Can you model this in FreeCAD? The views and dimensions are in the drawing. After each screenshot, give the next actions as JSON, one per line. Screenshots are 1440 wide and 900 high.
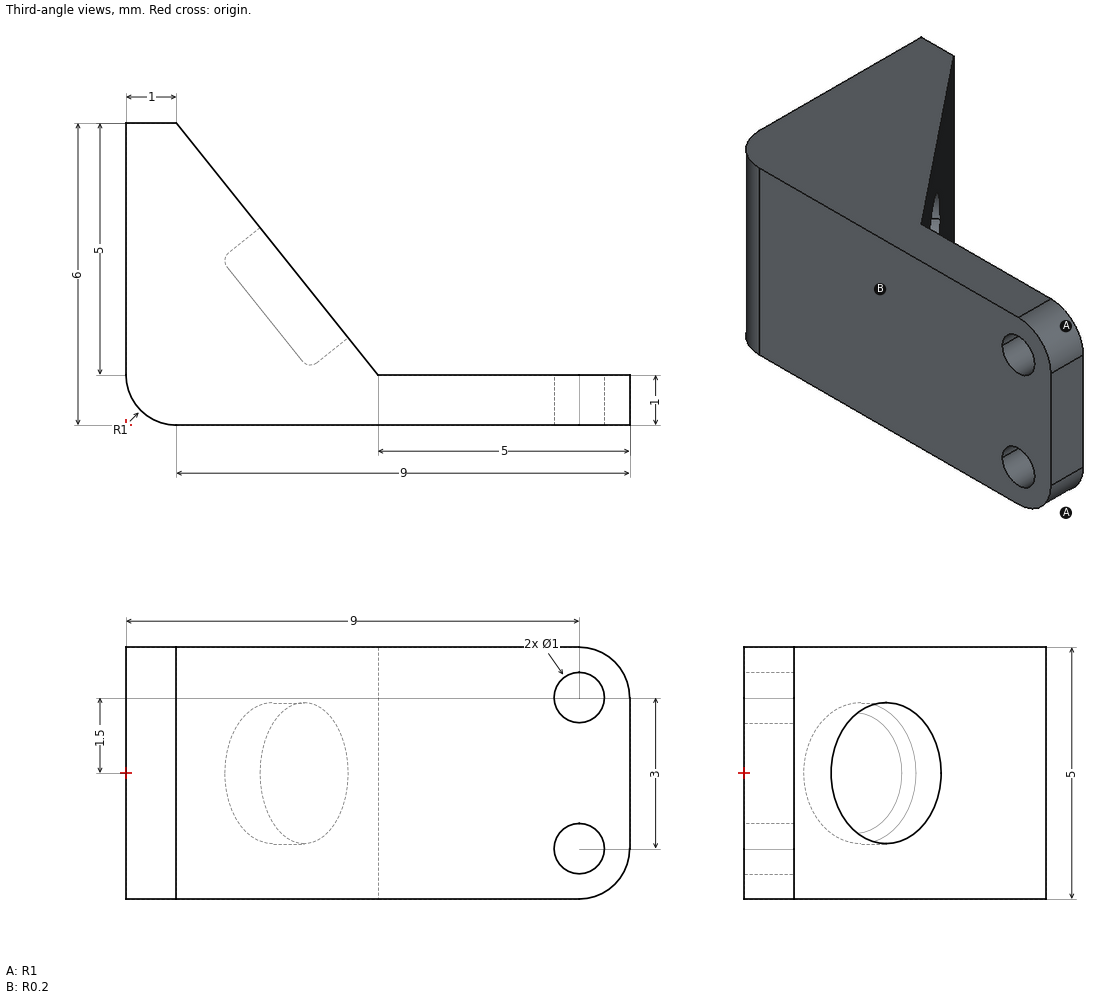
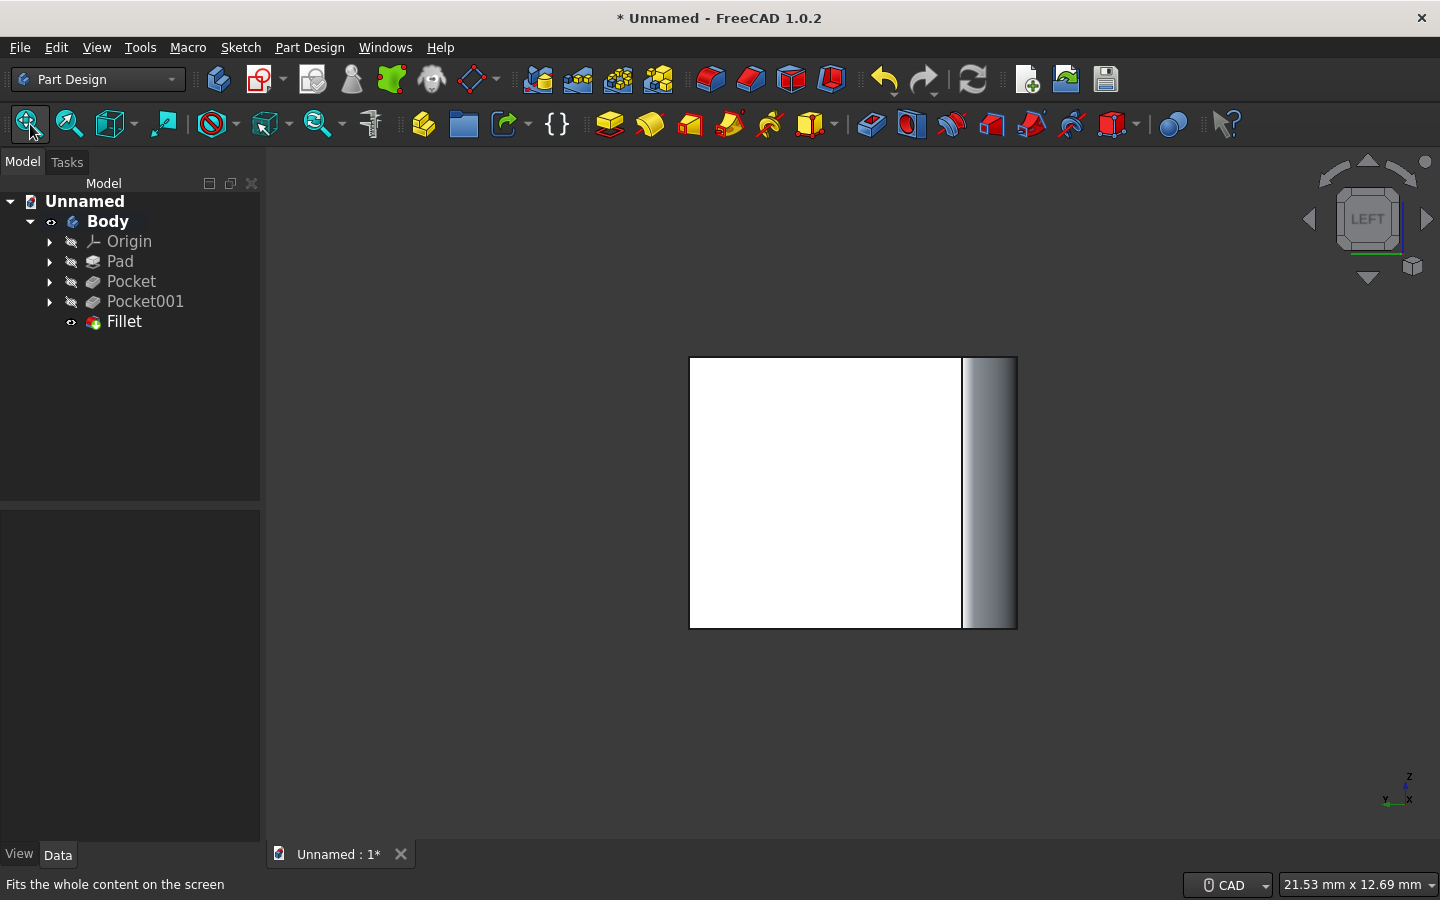
{"action": "key", "text": "v f"}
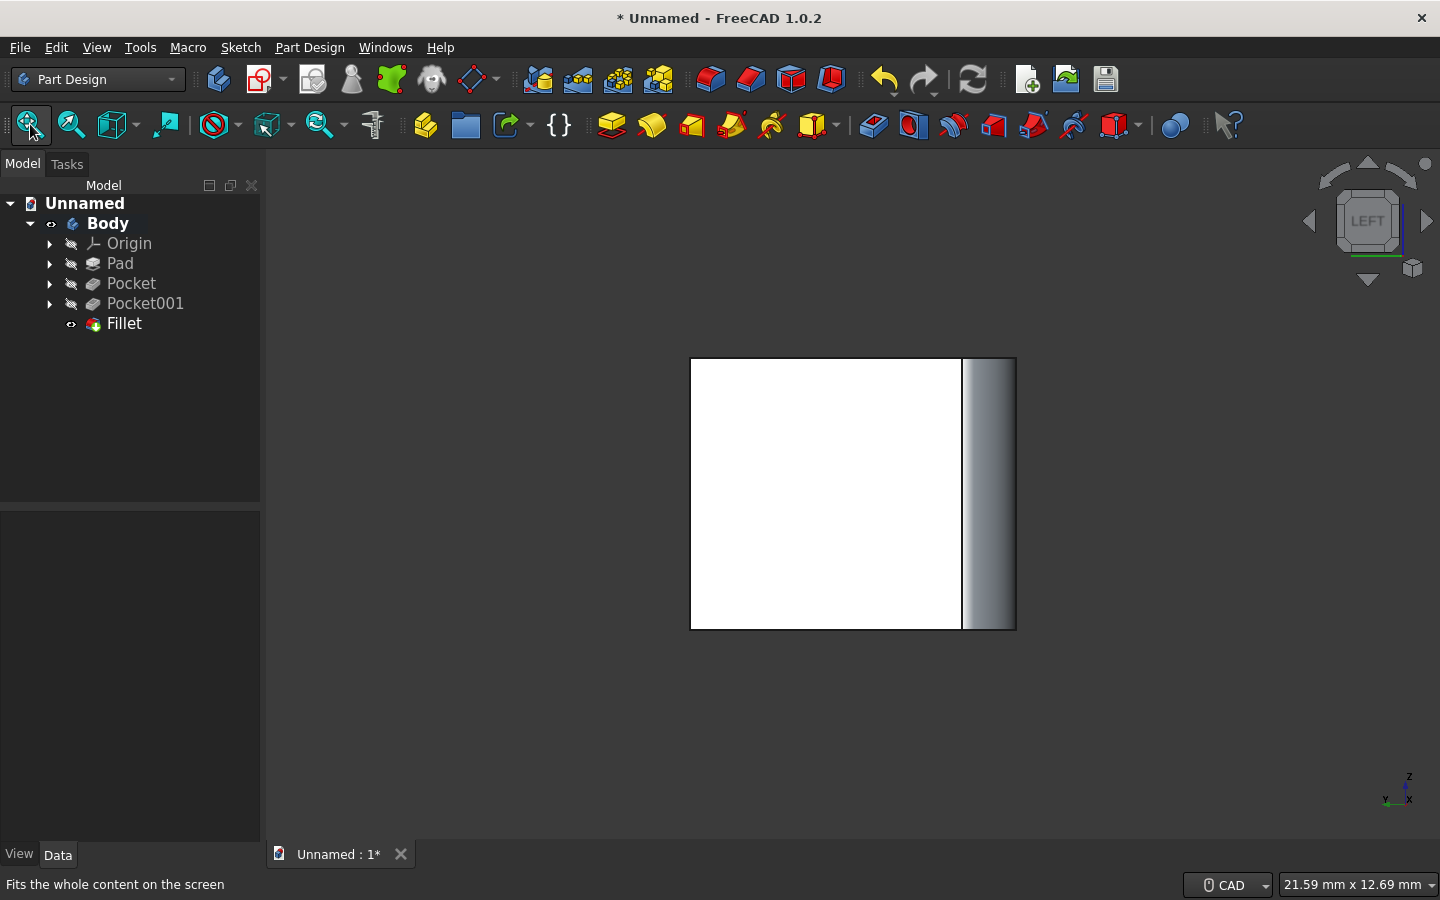
{"action": "key", "text": "v 3"}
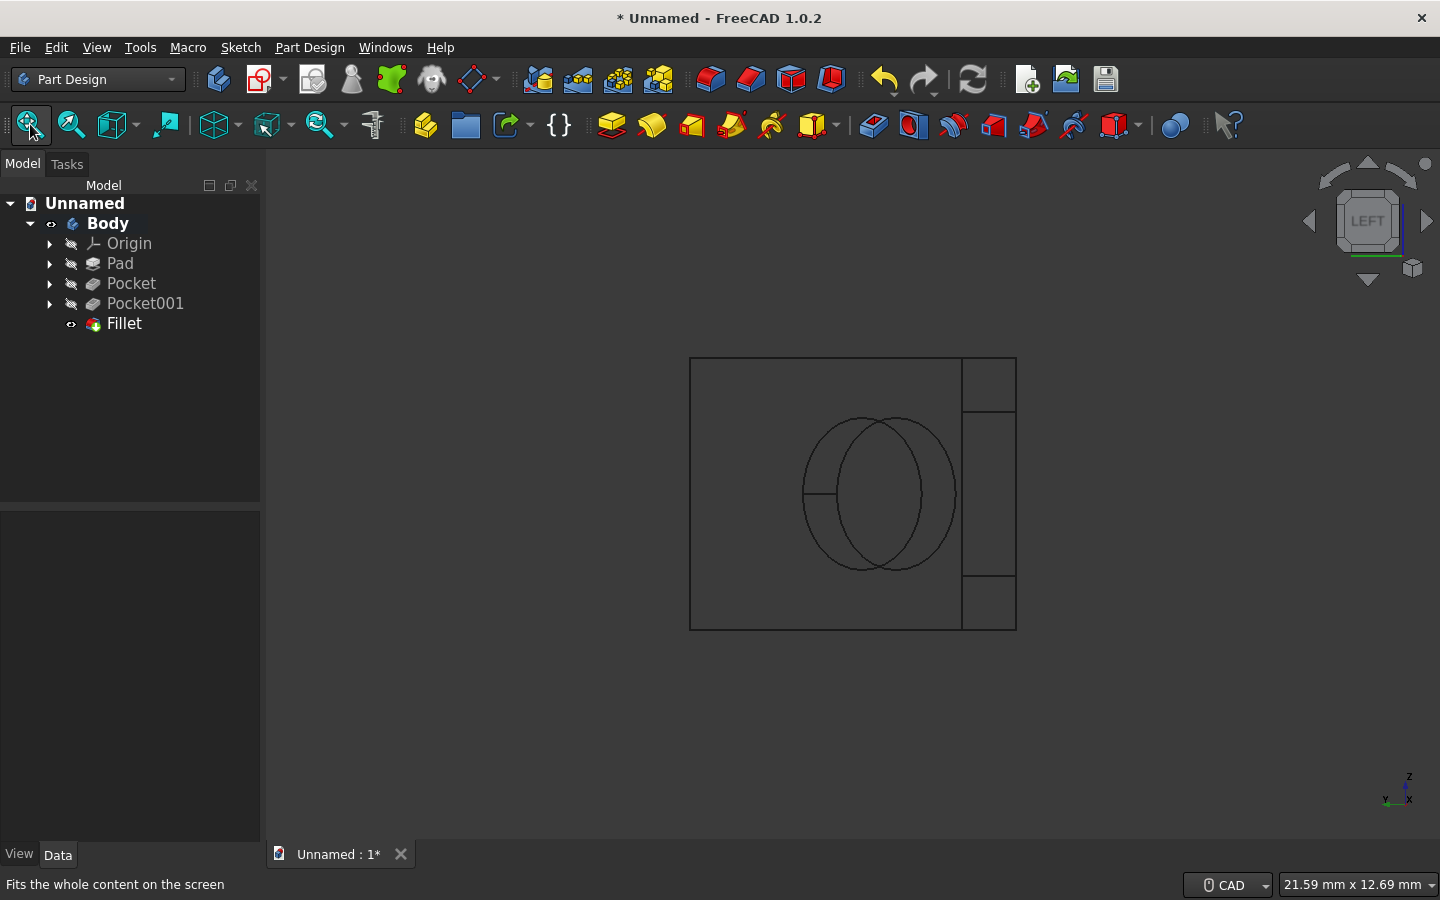
{"action": "key", "text": "0"}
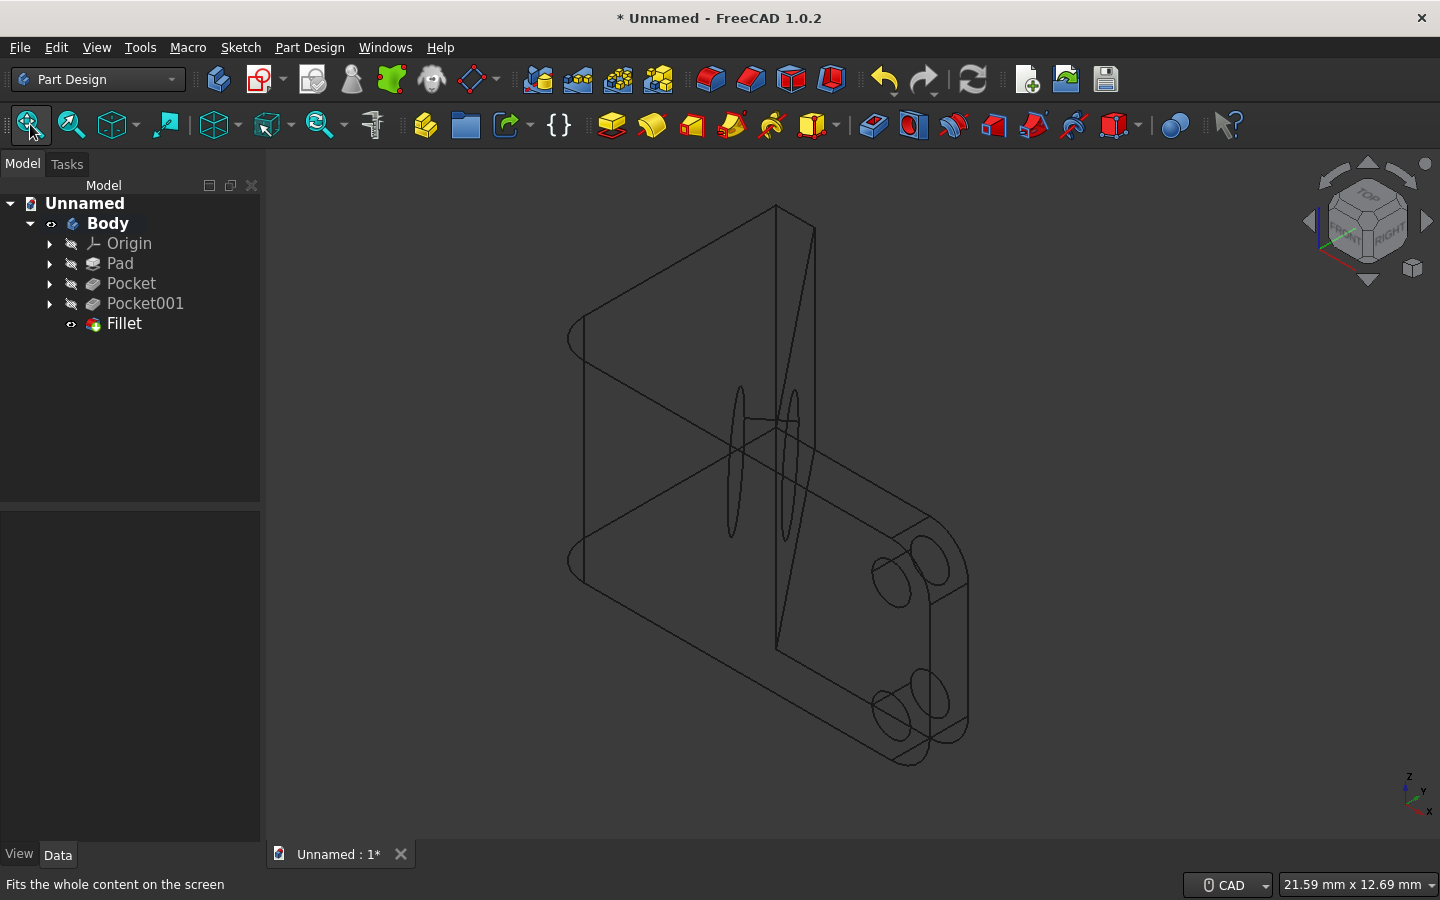
{"action": "left_click", "coordinate": [728, 505]}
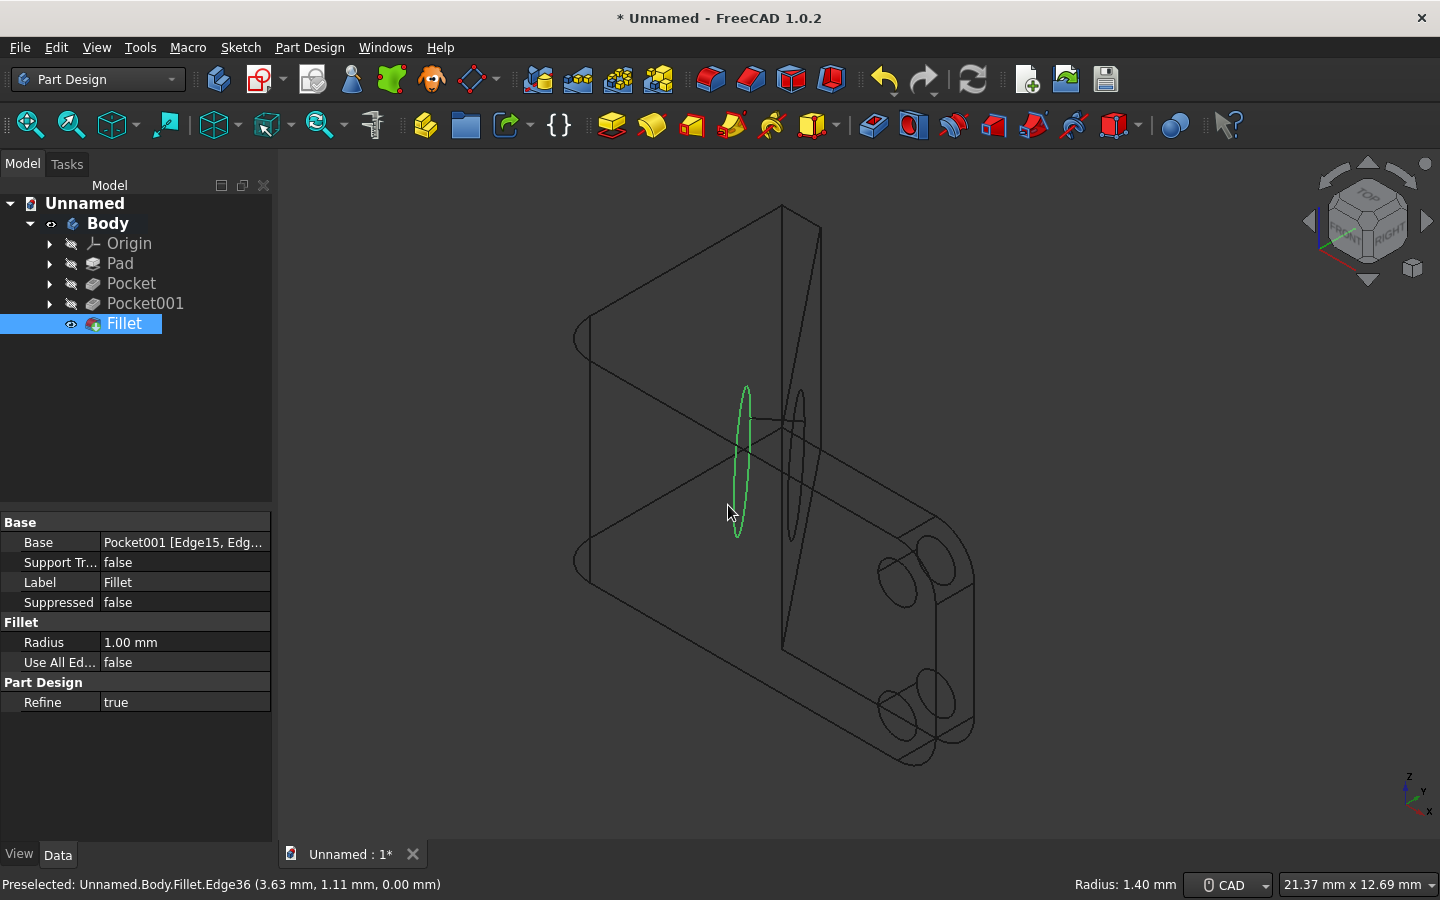
{"action": "key", "text": "v 1"}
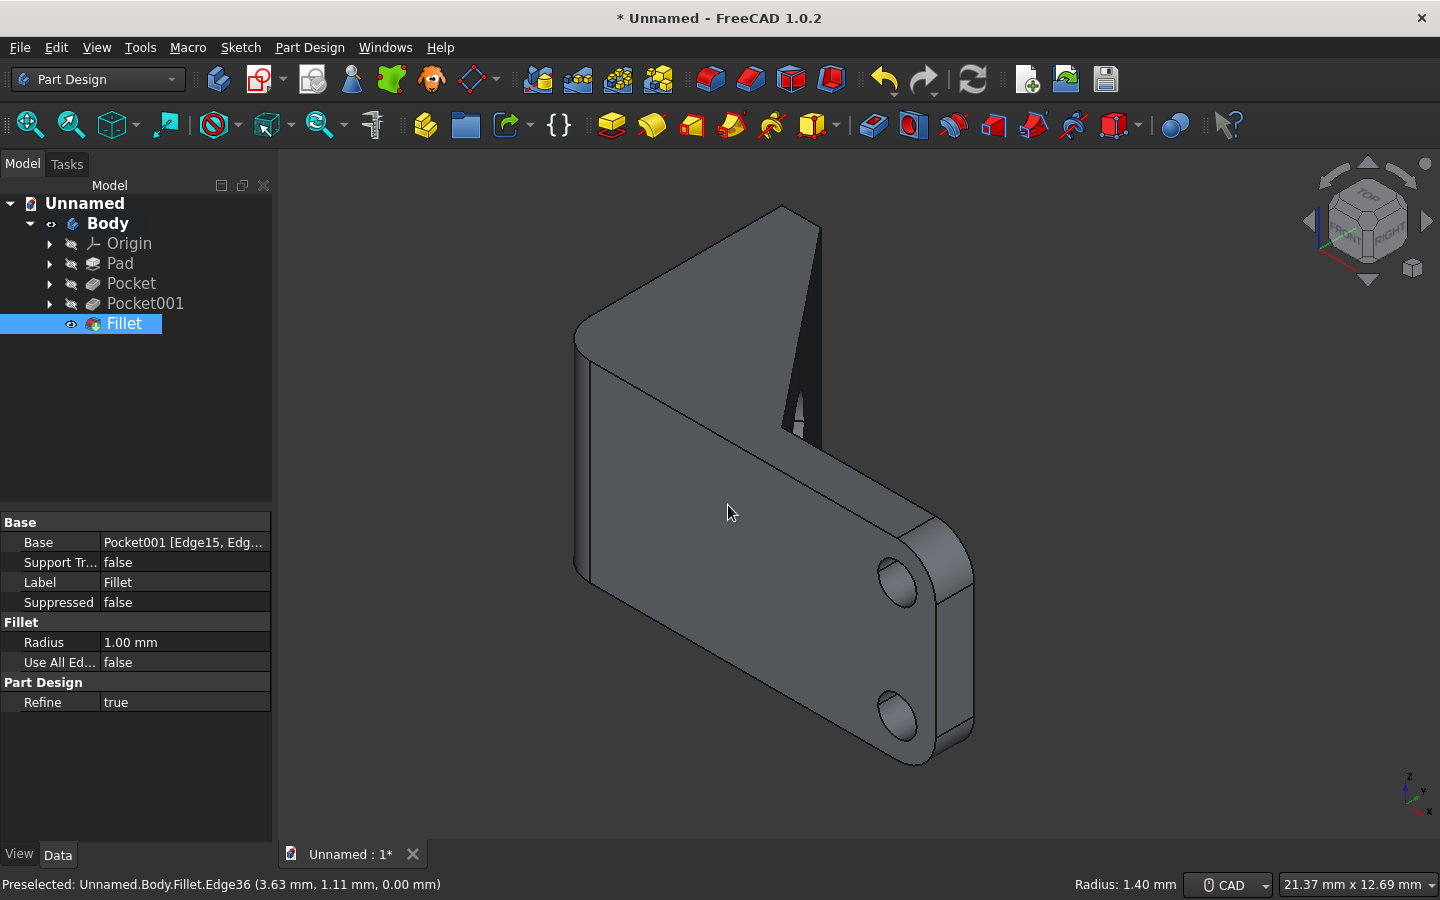
{"action": "left_click", "coordinate": [712, 80]}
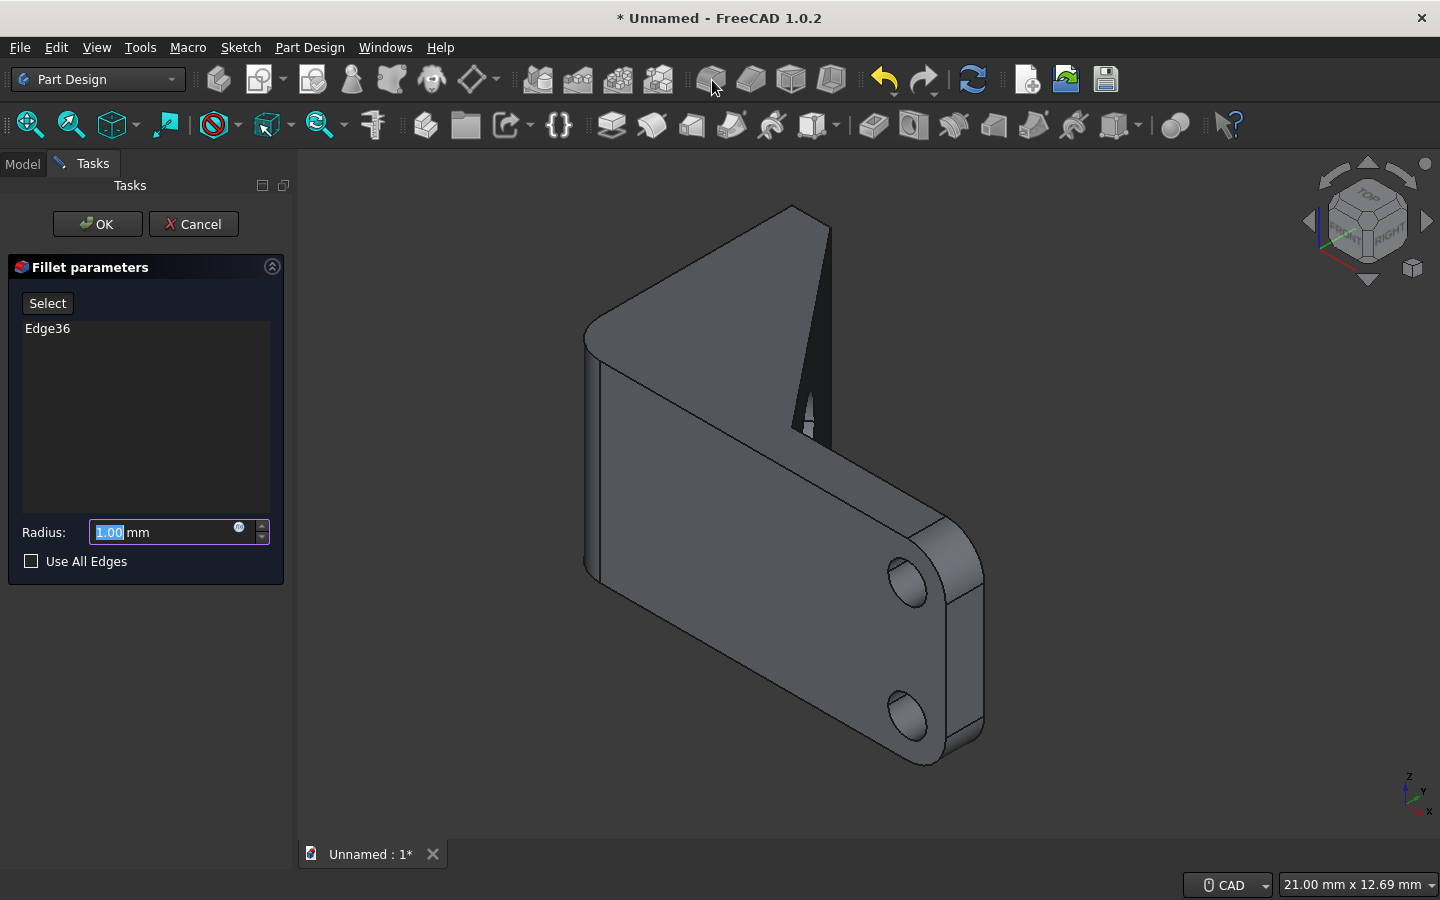
{"action": "type", "text": "0.2"}
{"action": "key", "text": "Tab"}